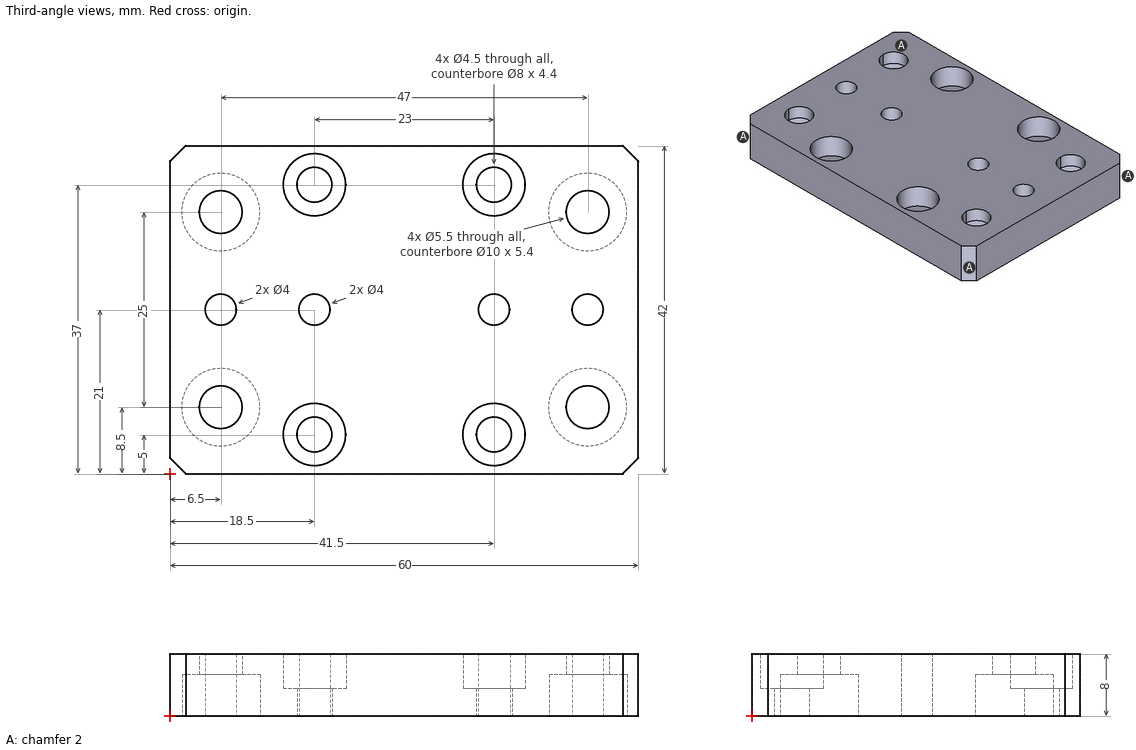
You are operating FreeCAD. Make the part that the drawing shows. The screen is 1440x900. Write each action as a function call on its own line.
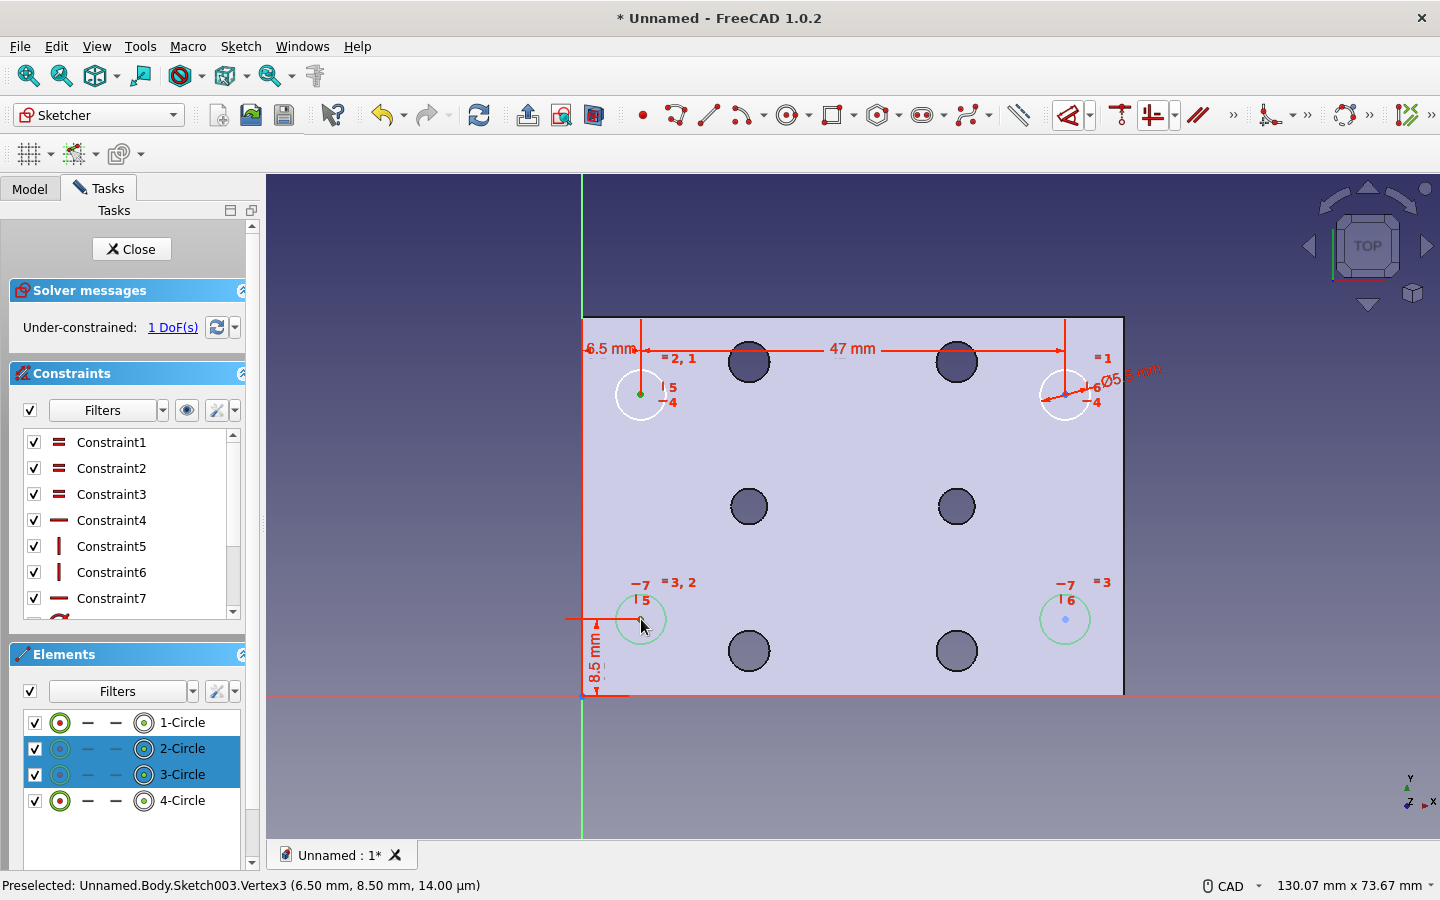
click(1090, 116)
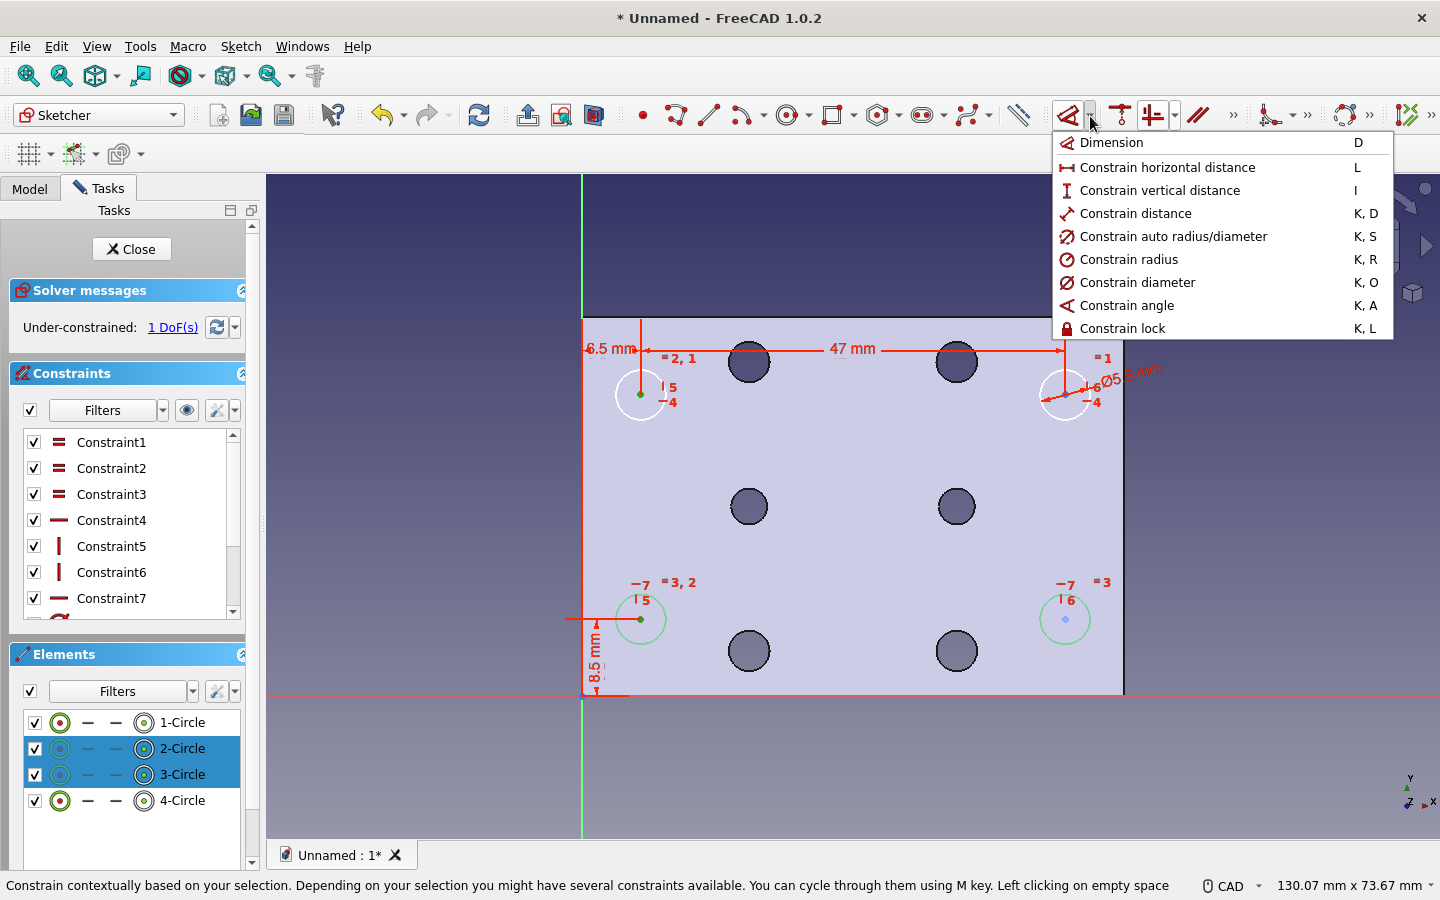
click(1223, 190)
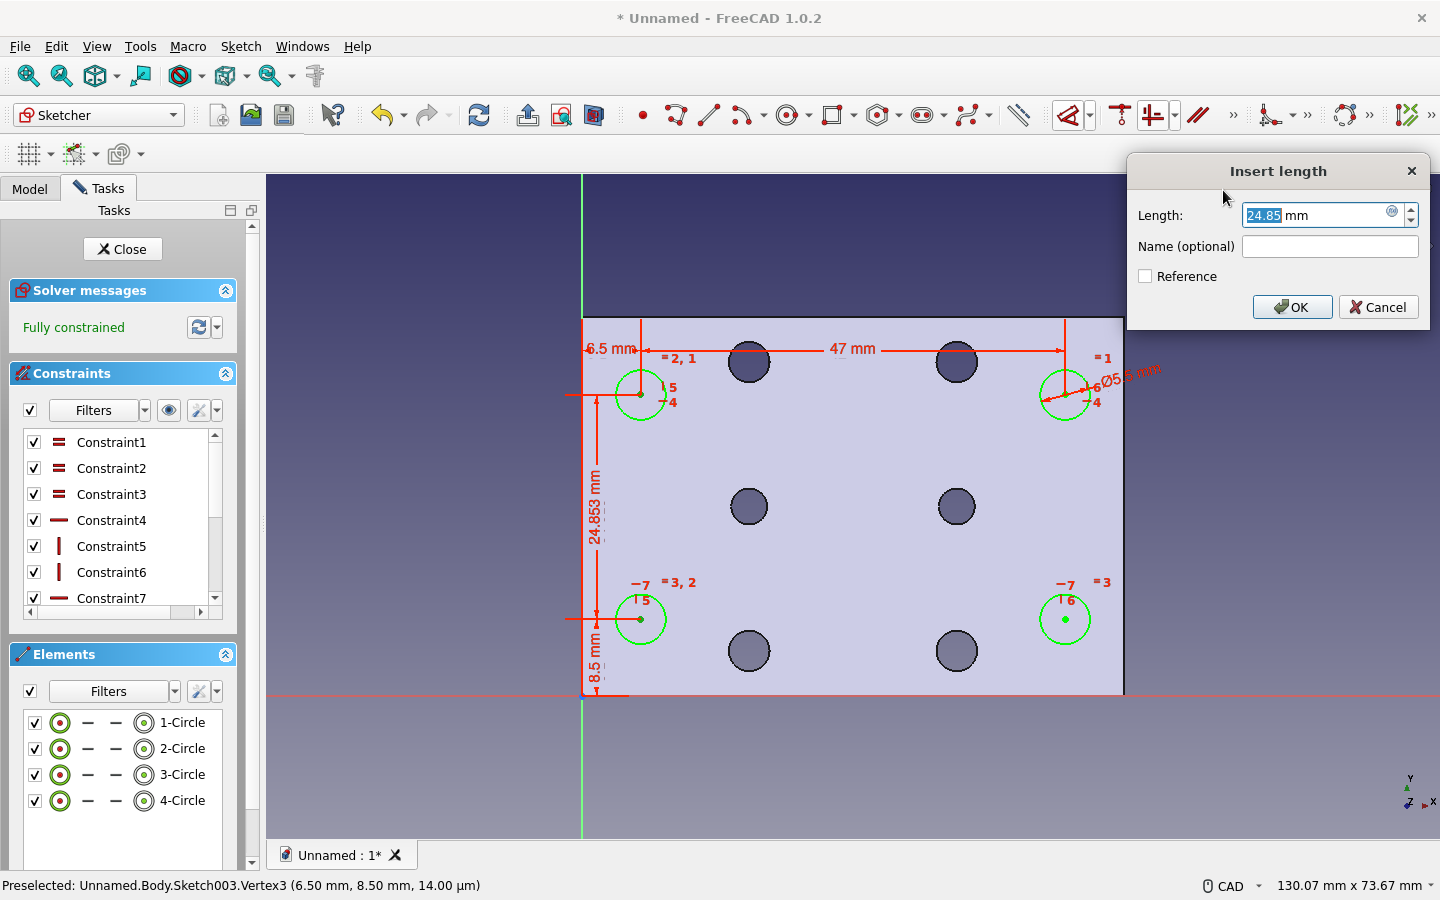
text(25)
key(Return)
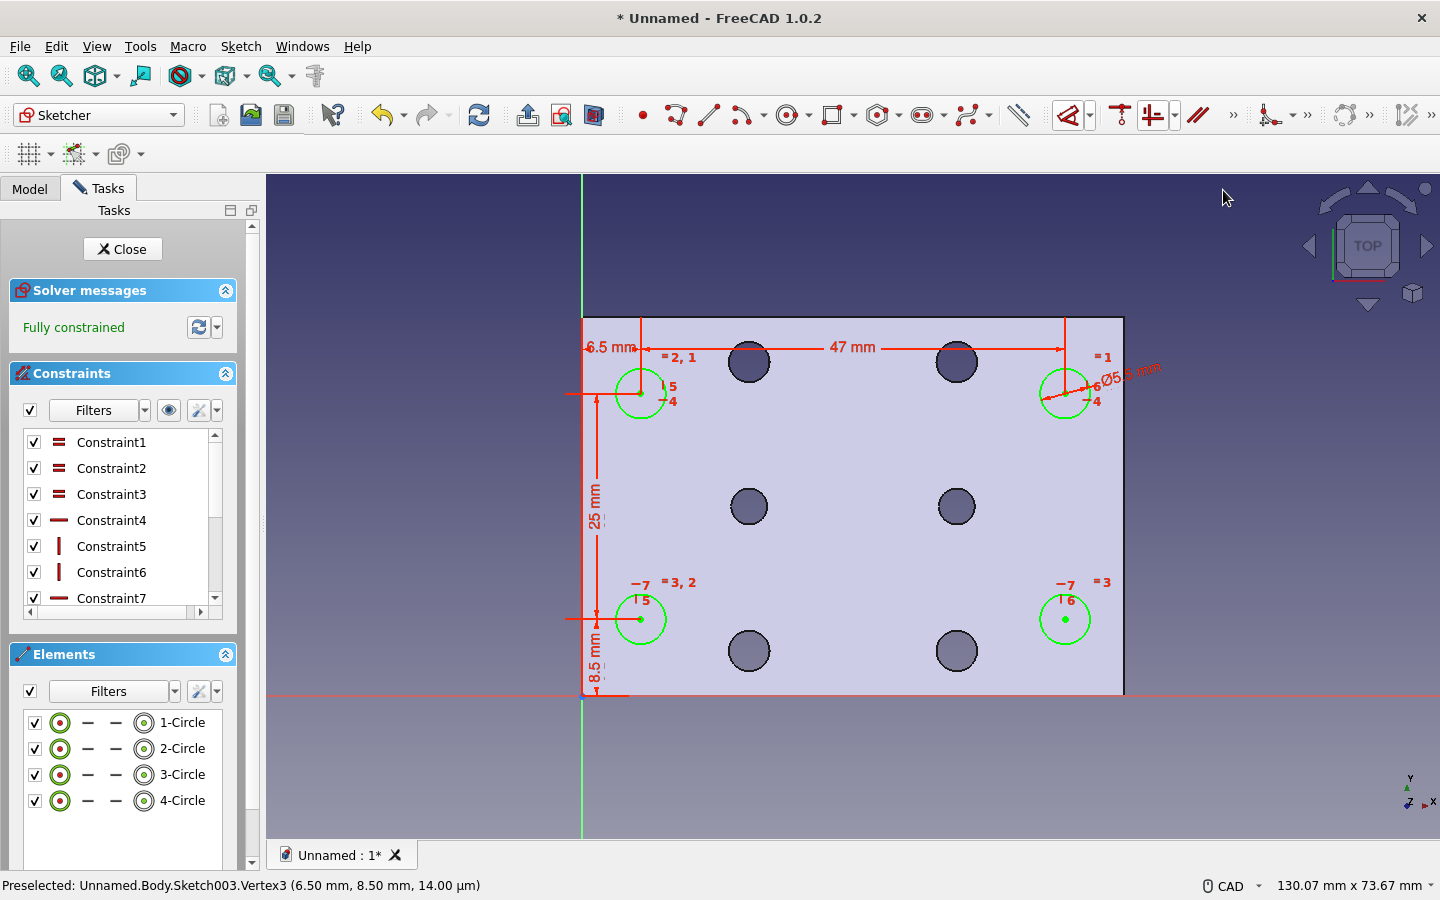
click(123, 249)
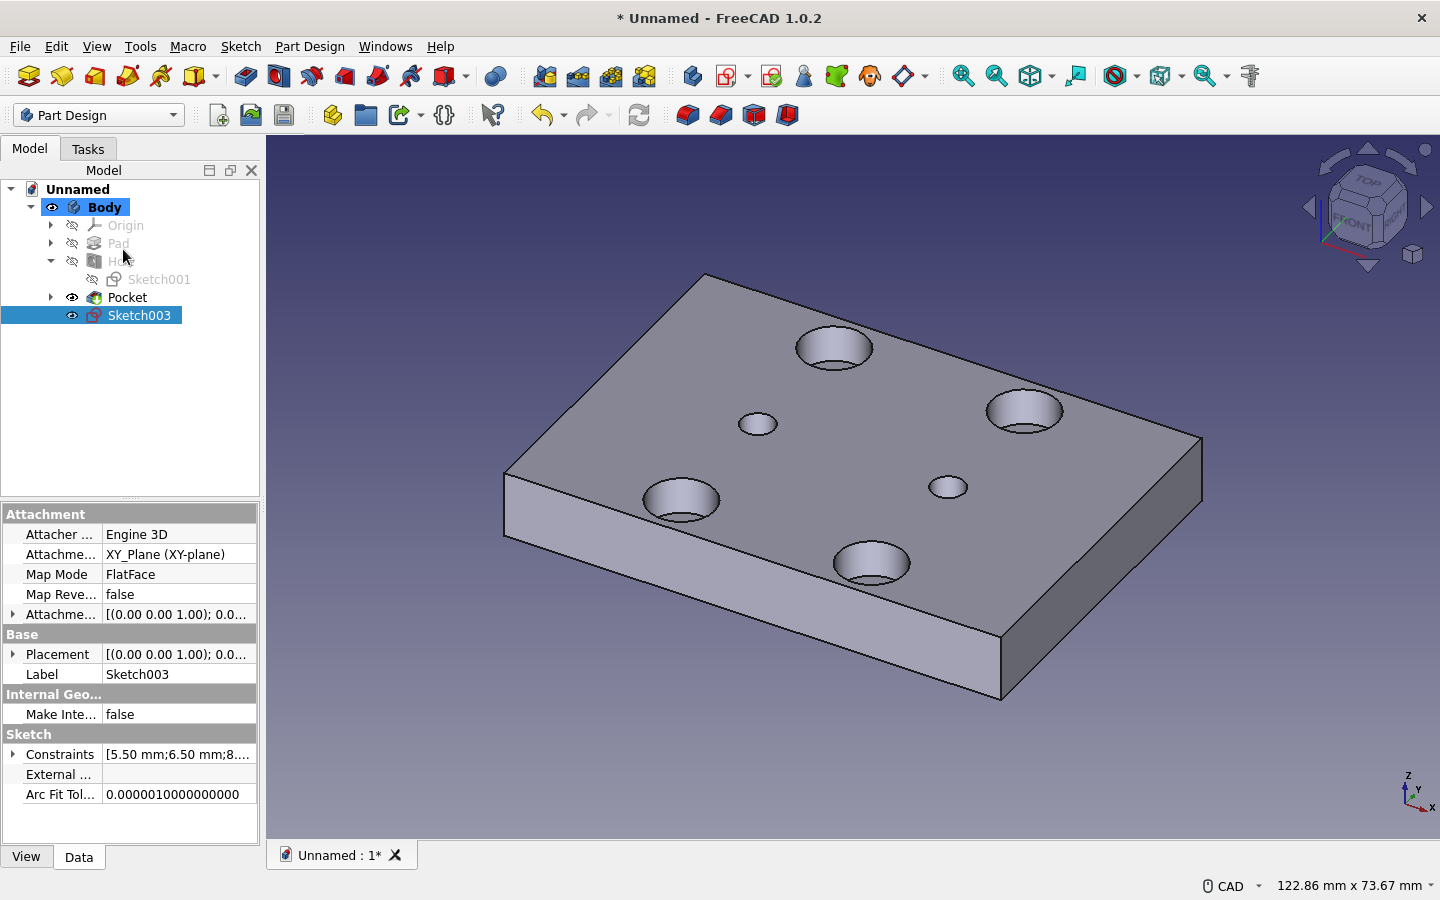
click(279, 76)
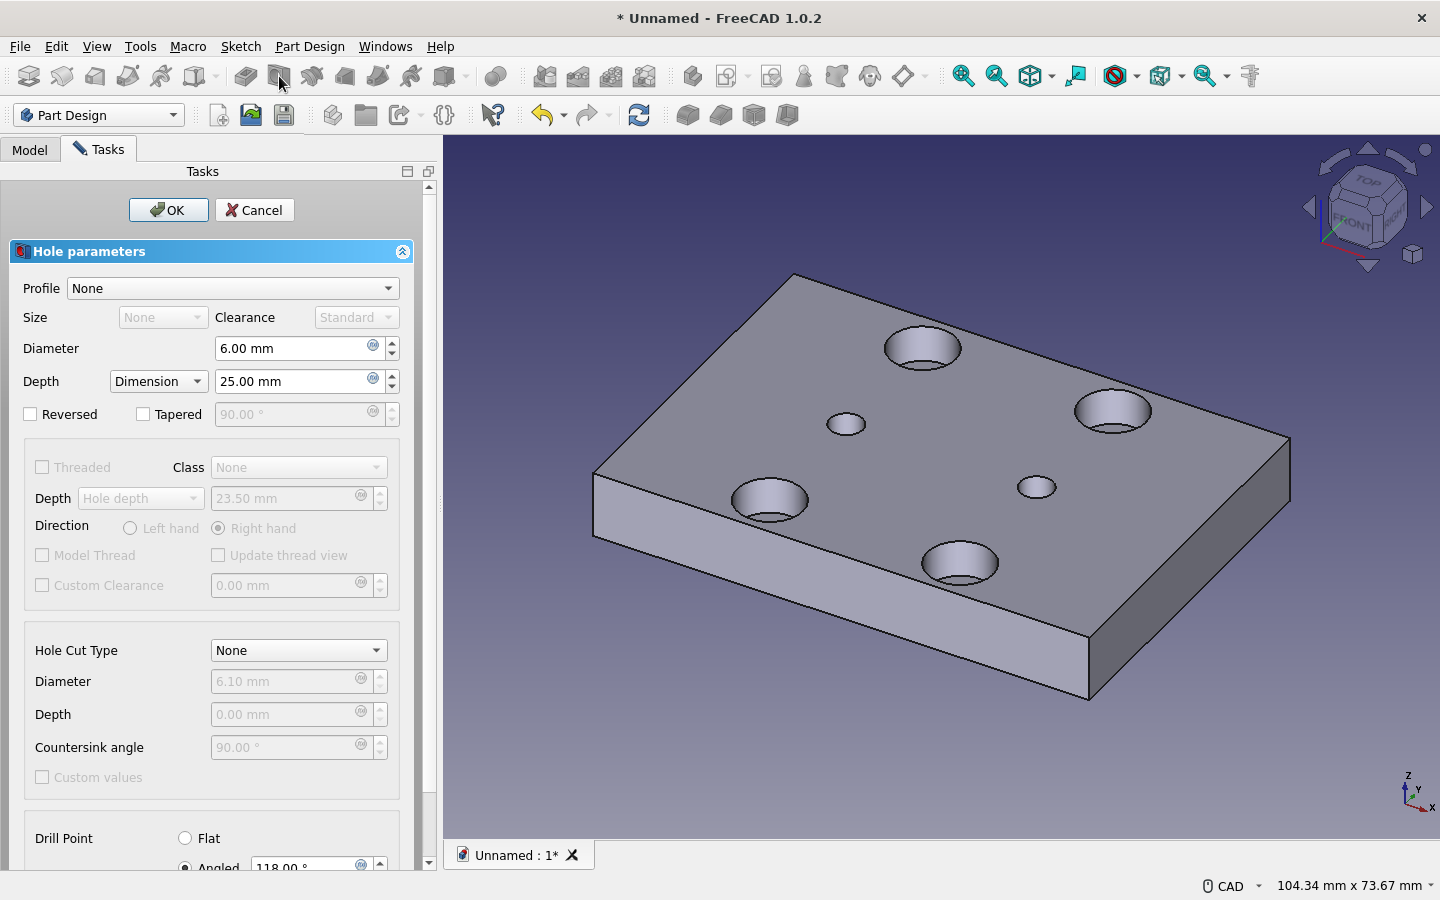
triple_click(300, 348)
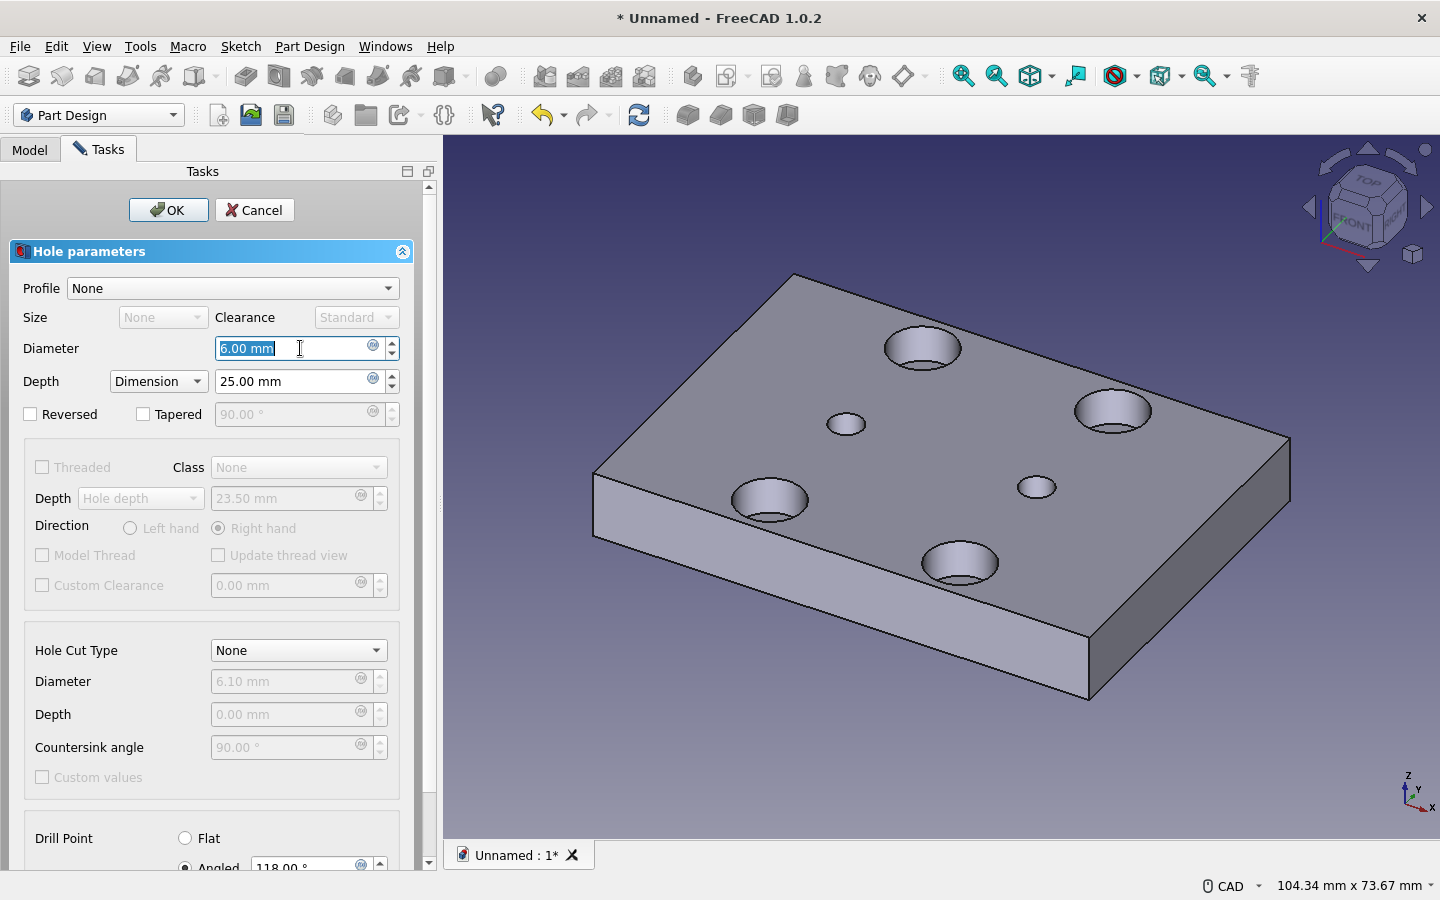
text(5.5)
key(Tab)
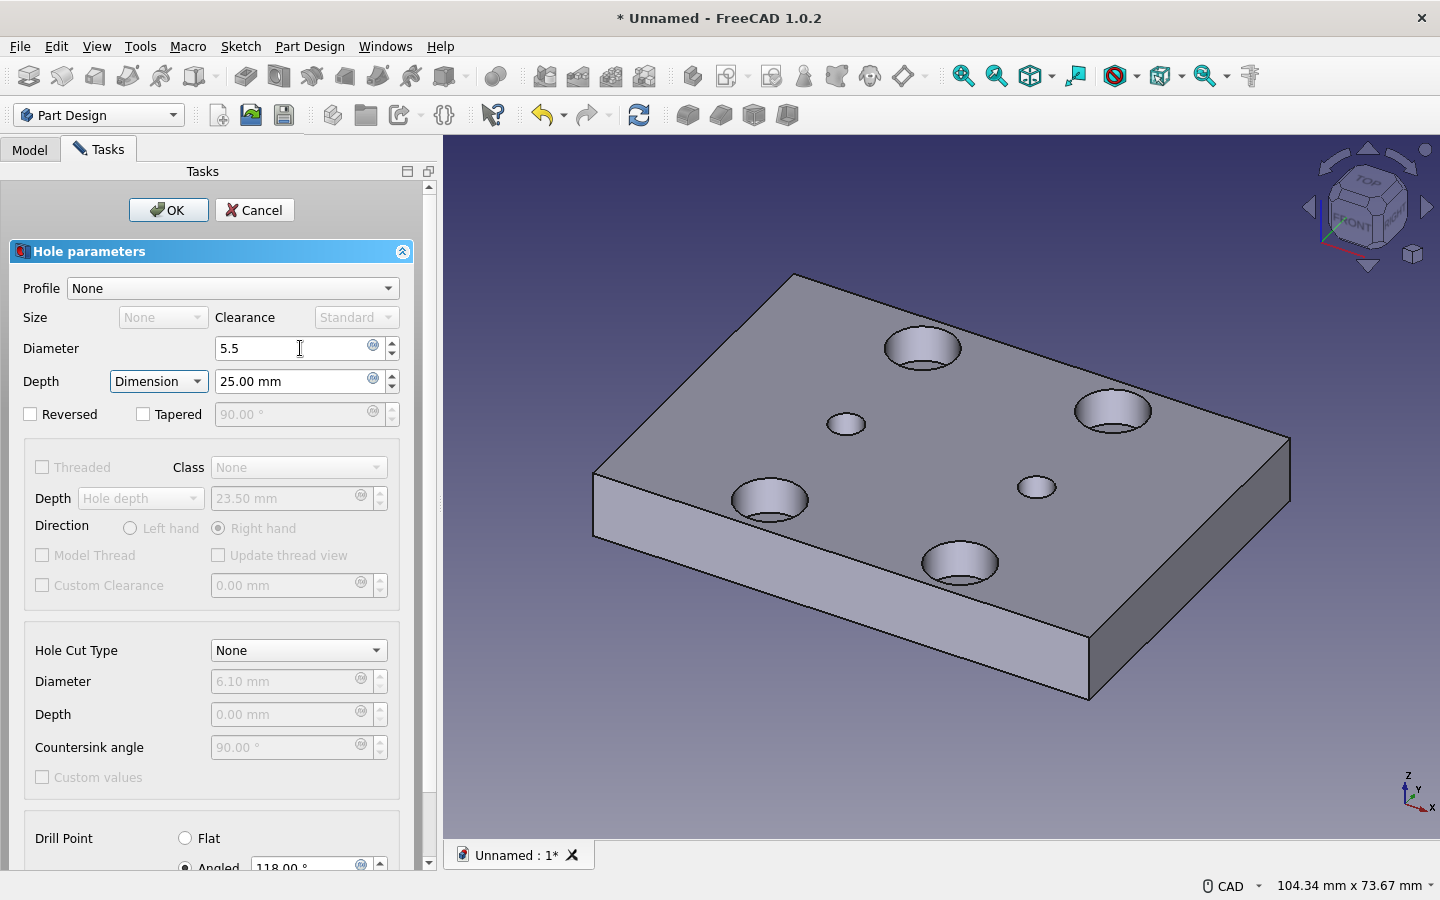
click(160, 382)